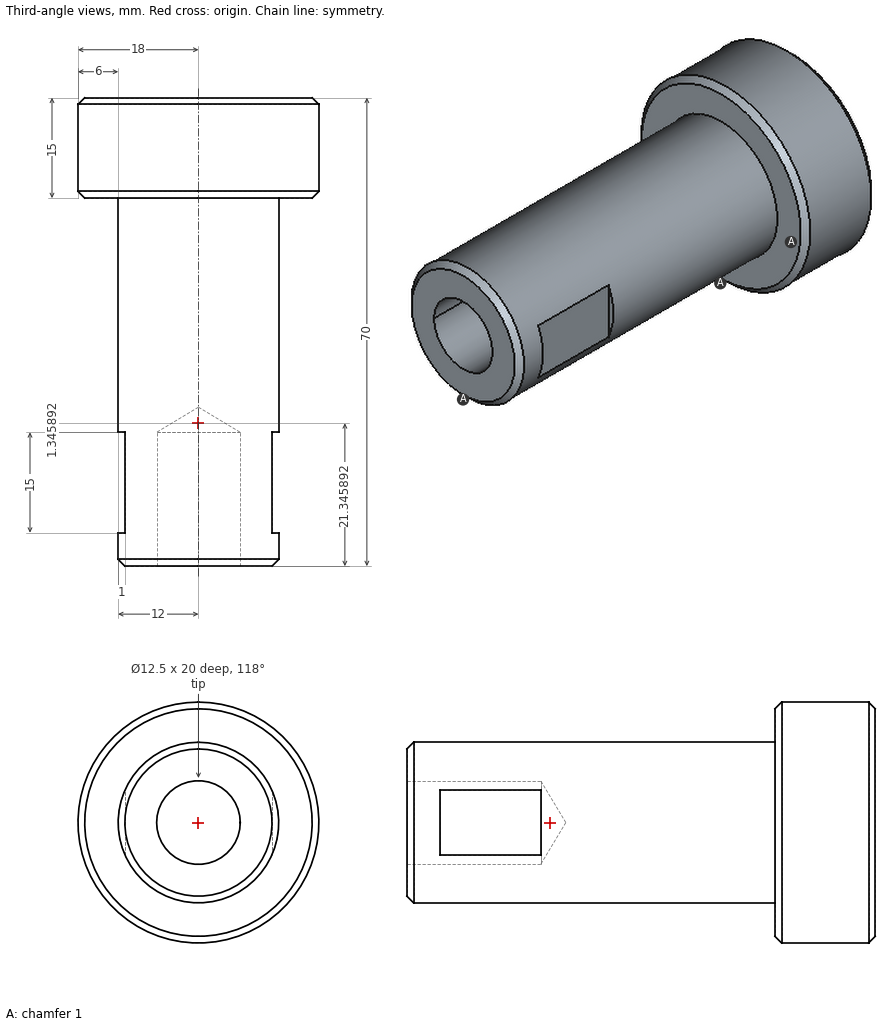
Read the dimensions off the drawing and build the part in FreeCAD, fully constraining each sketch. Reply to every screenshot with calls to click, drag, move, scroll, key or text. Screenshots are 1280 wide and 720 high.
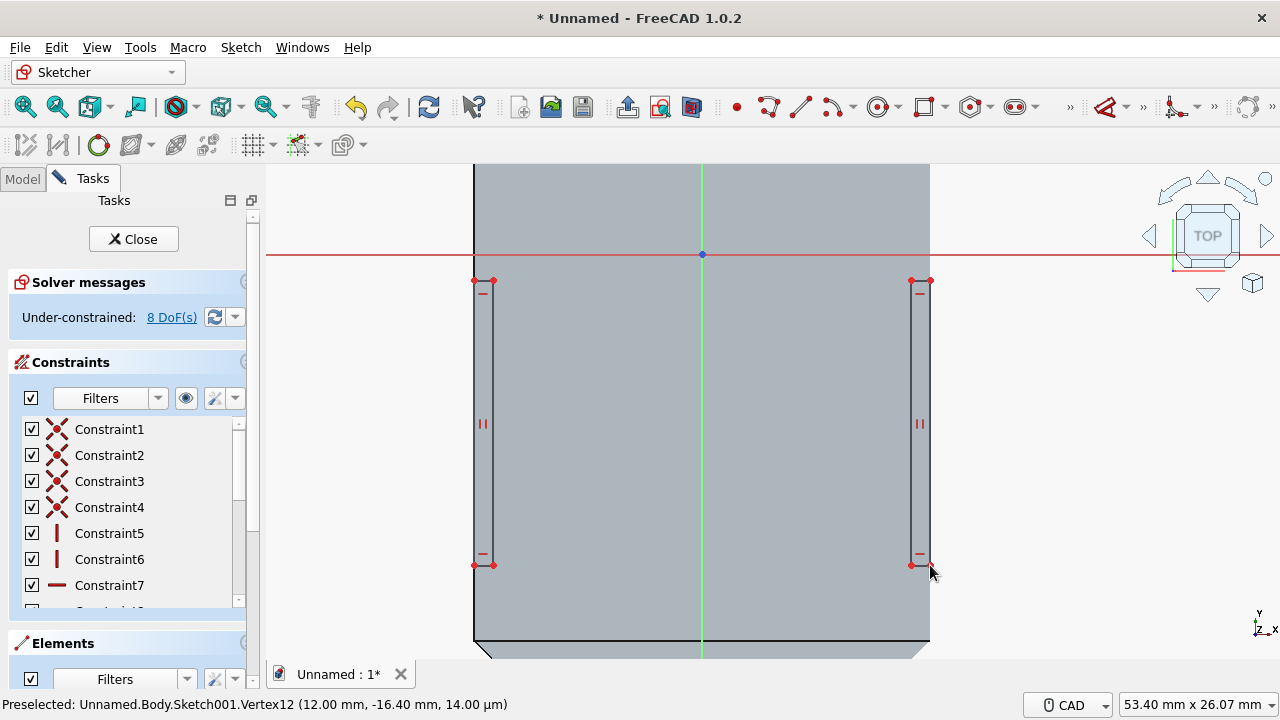
click(493, 281)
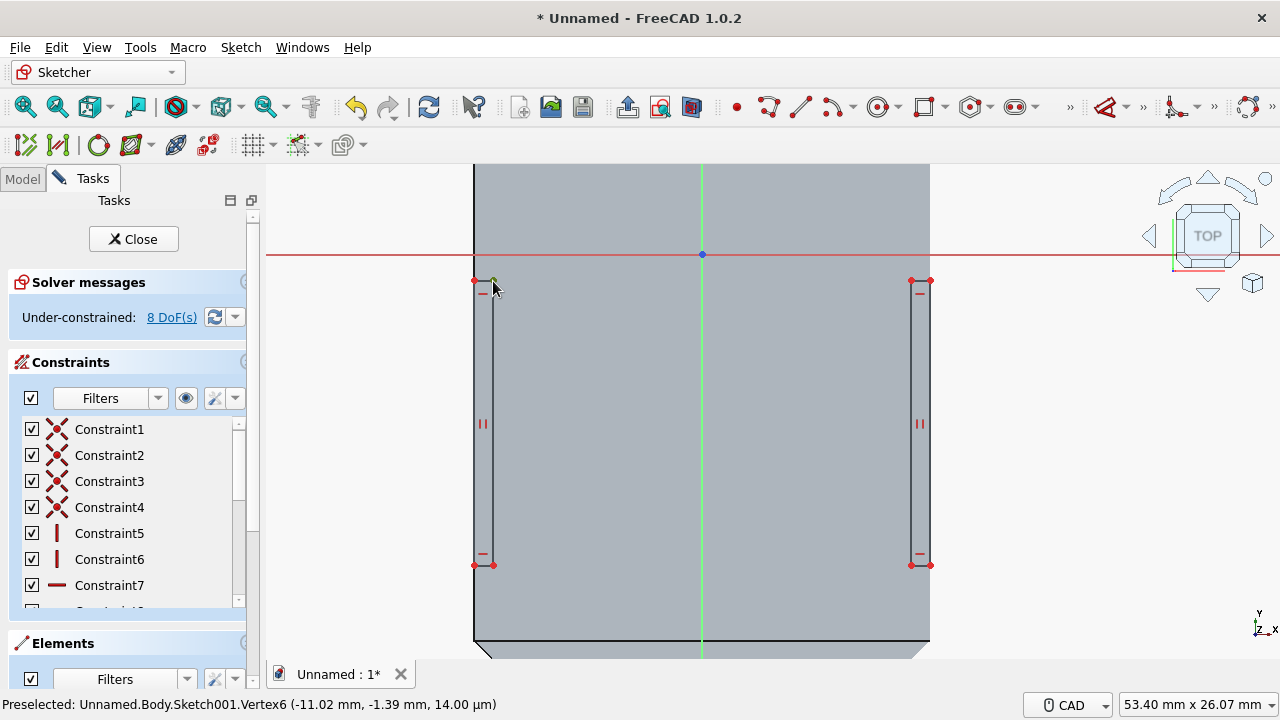
click(911, 281)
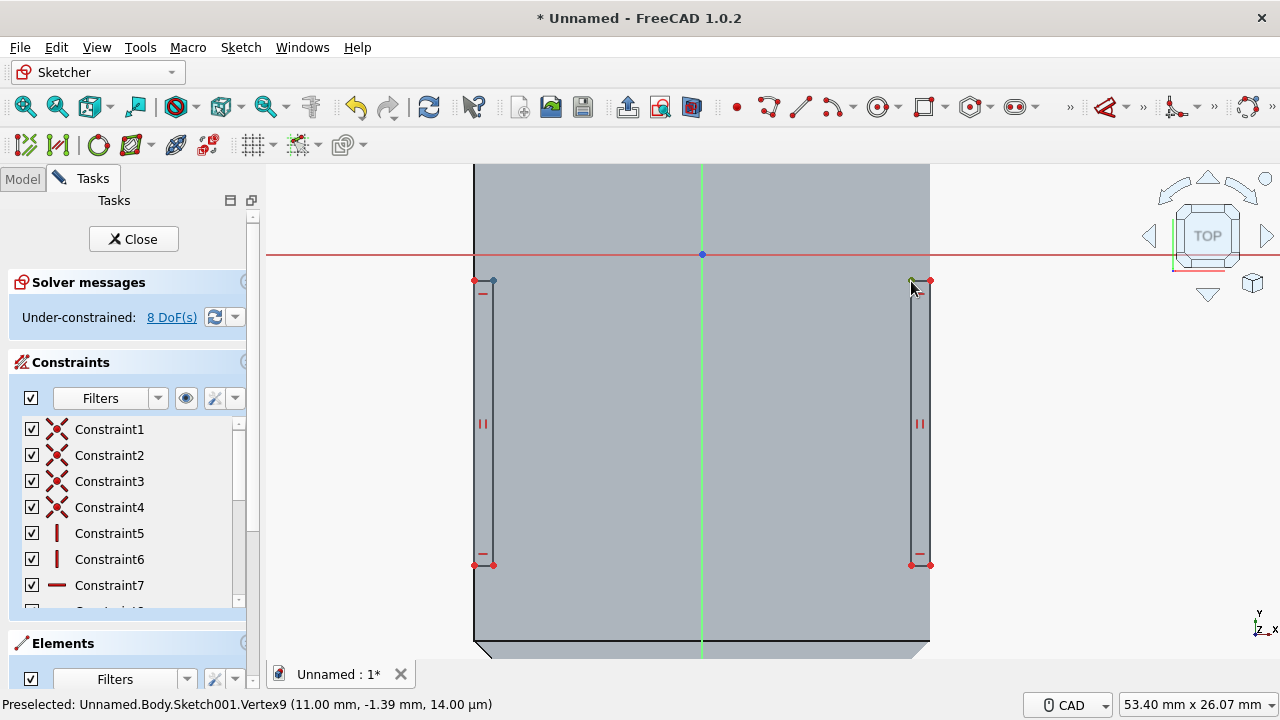
click(702, 600)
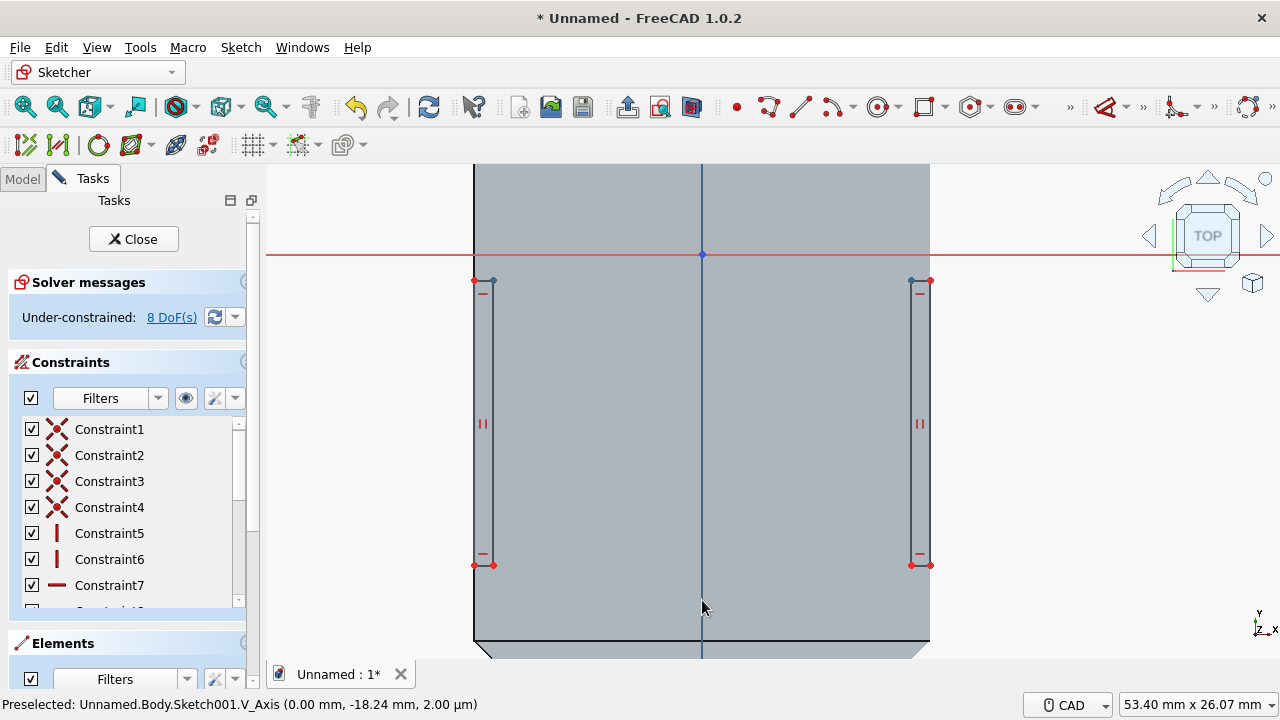
key(s)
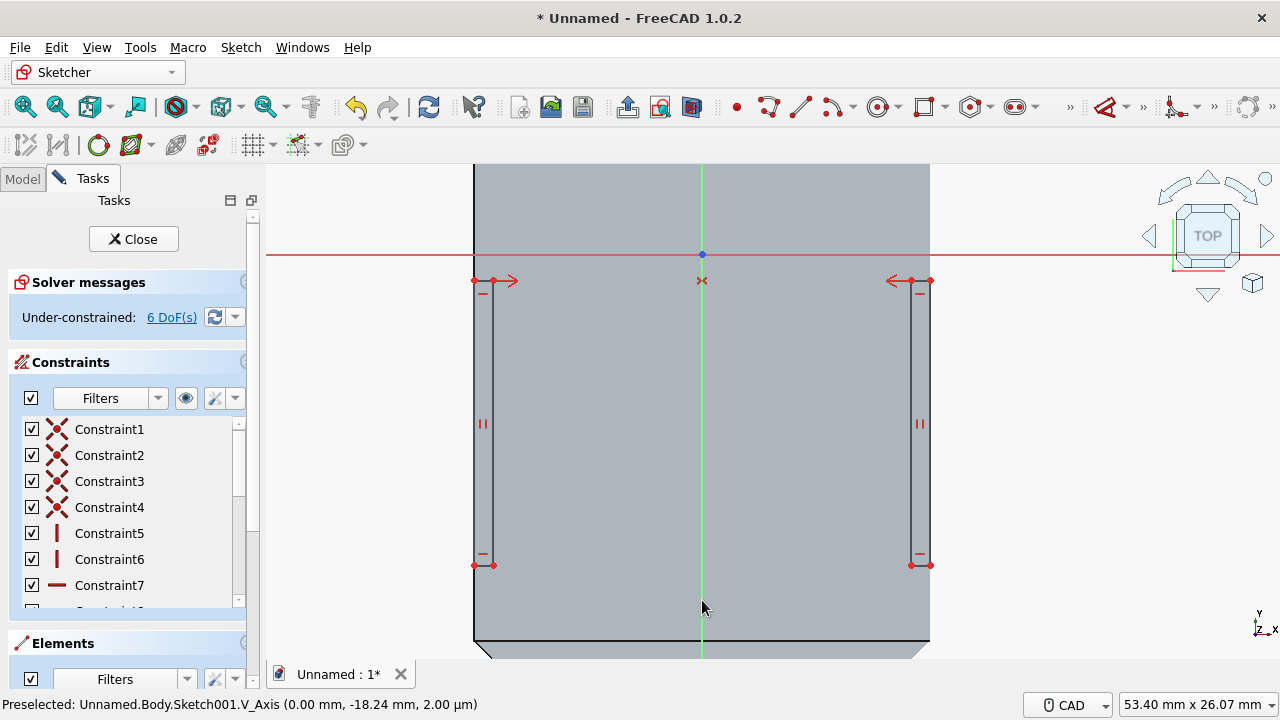
click(474, 566)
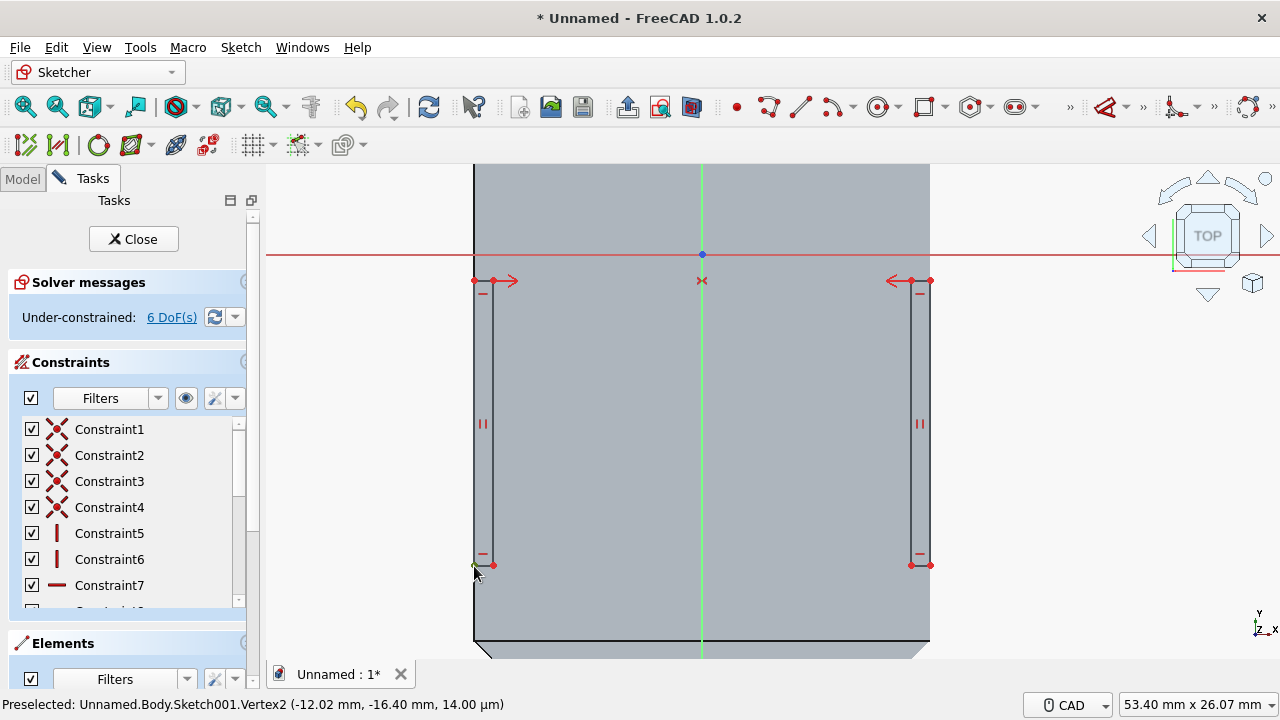
click(930, 566)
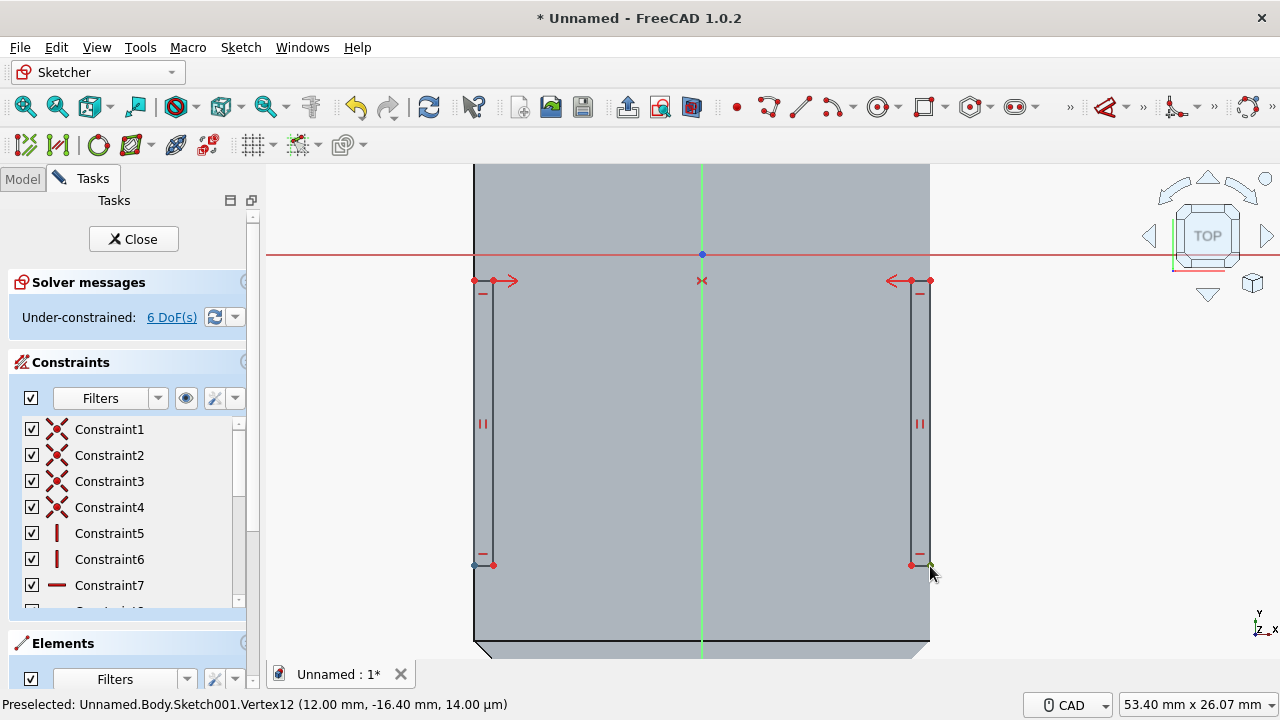
click(702, 600)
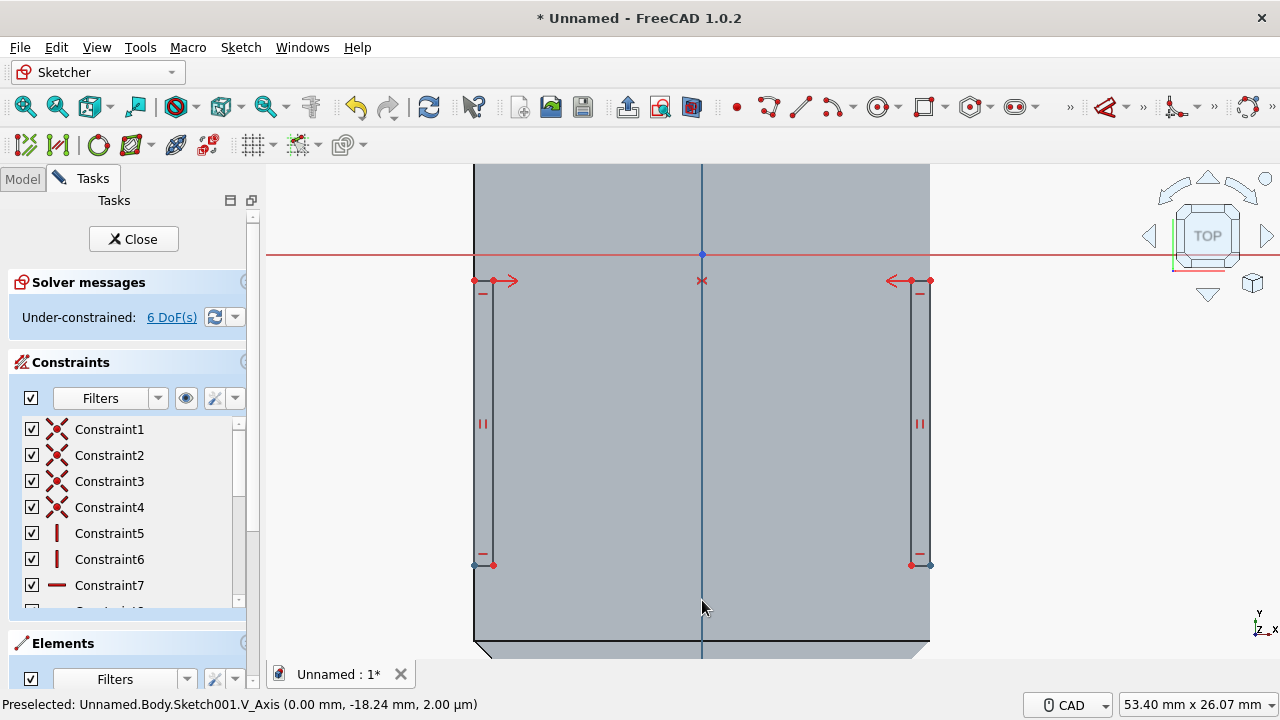
key(s)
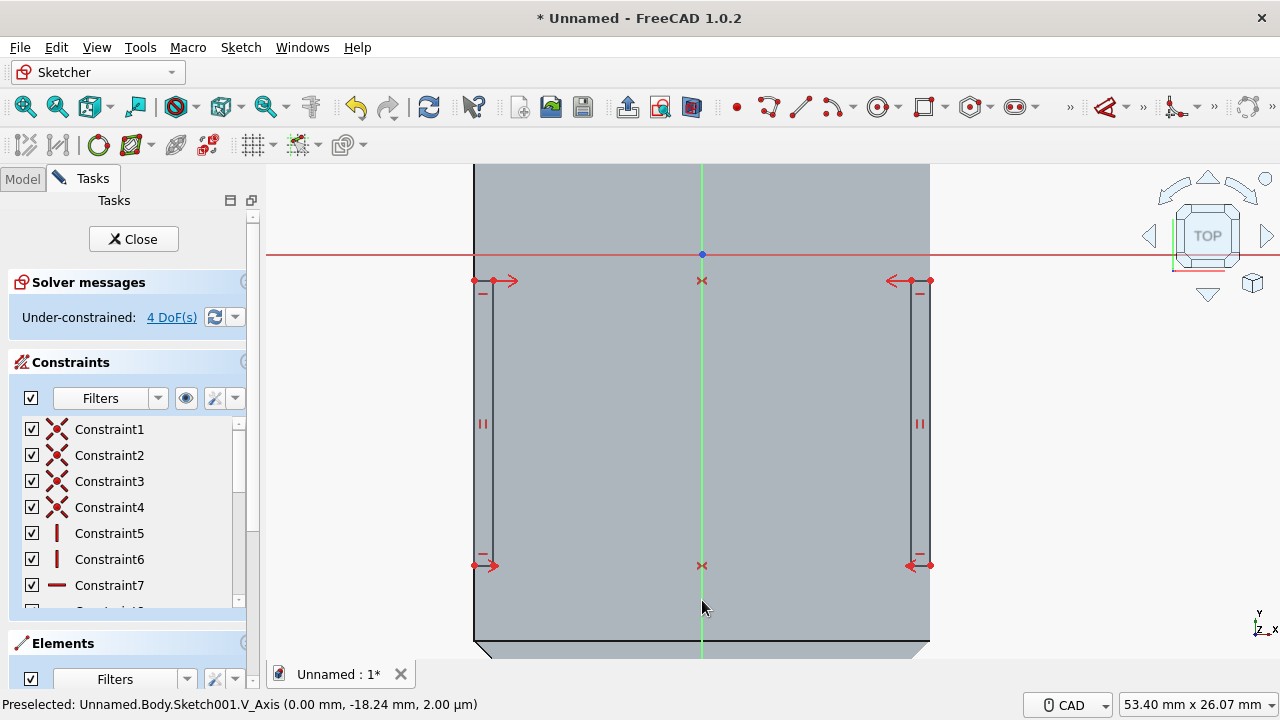
click(1106, 108)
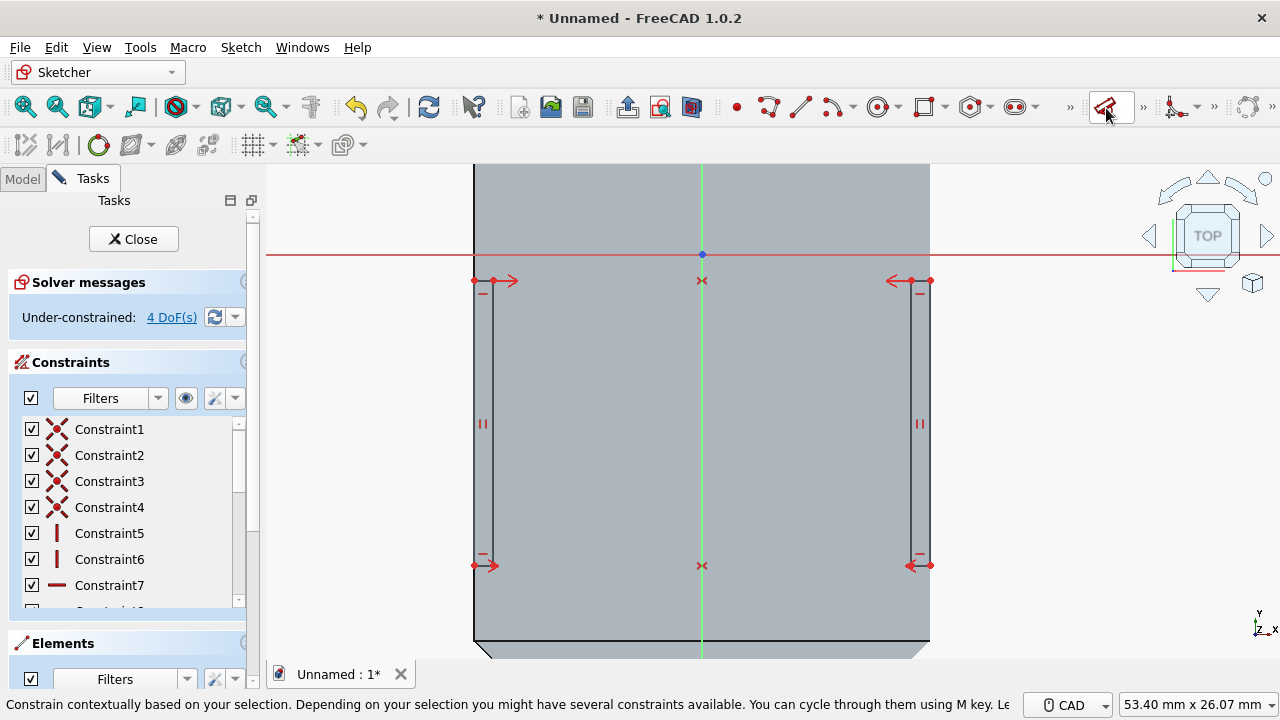
scroll(484, 566, up, 4)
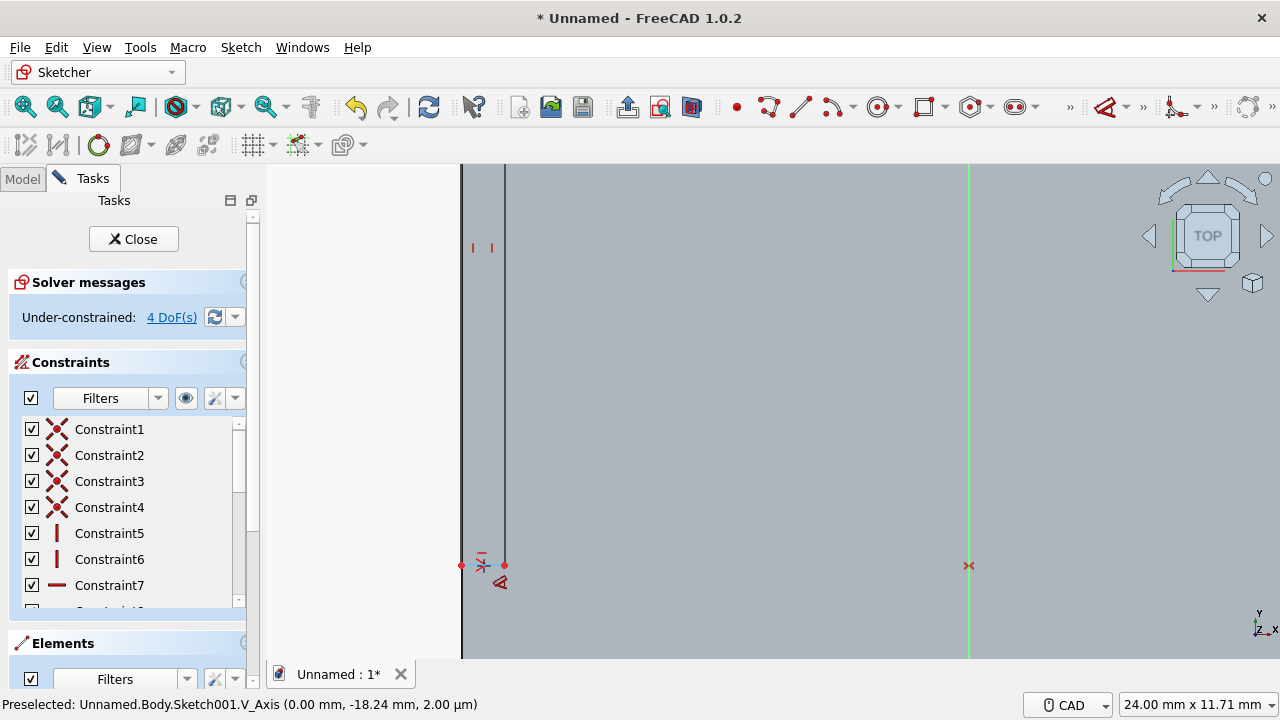
click(483, 565)
click(483, 599)